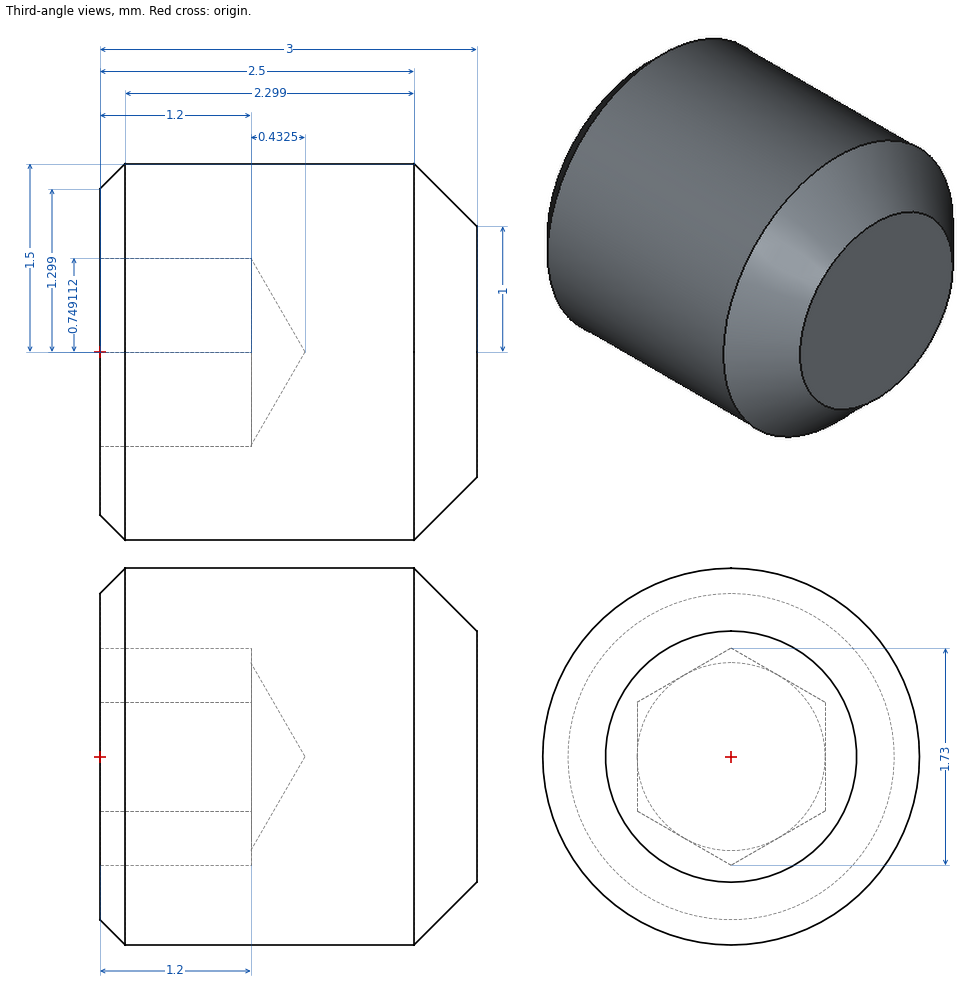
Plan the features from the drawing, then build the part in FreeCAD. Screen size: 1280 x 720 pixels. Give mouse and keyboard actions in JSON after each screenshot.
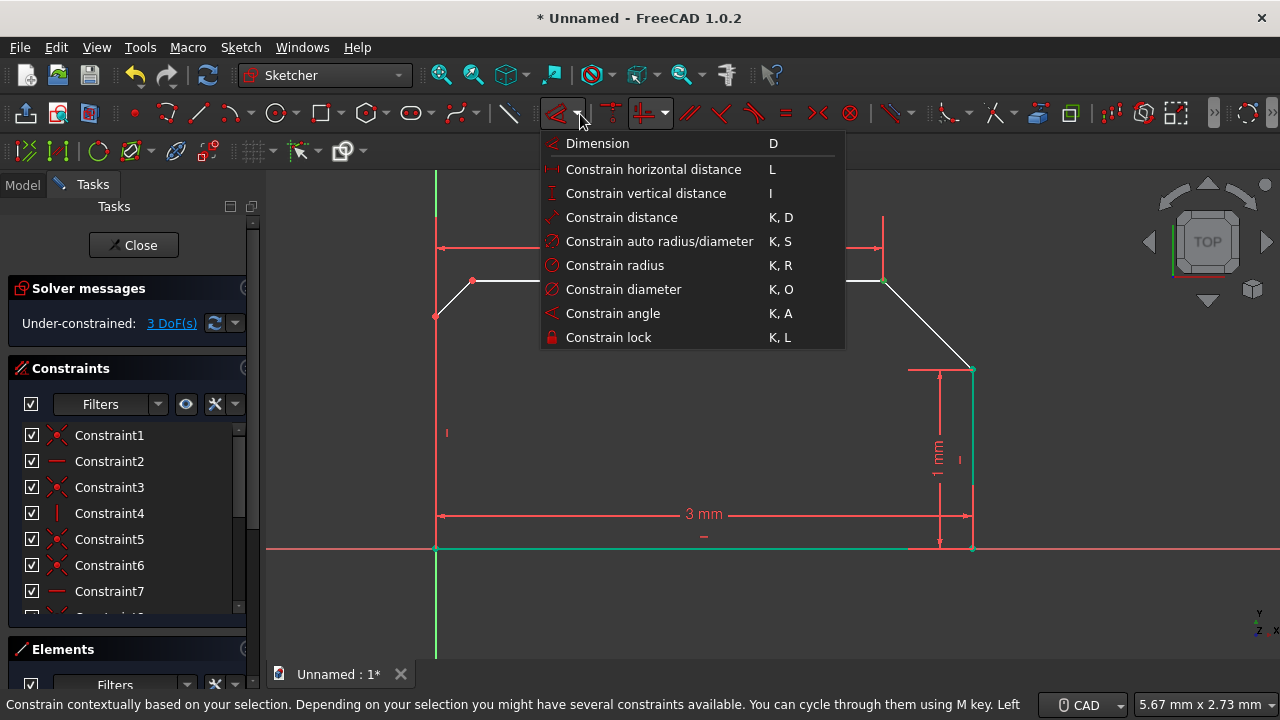
{"action": "left_click", "coordinate": [693, 193]}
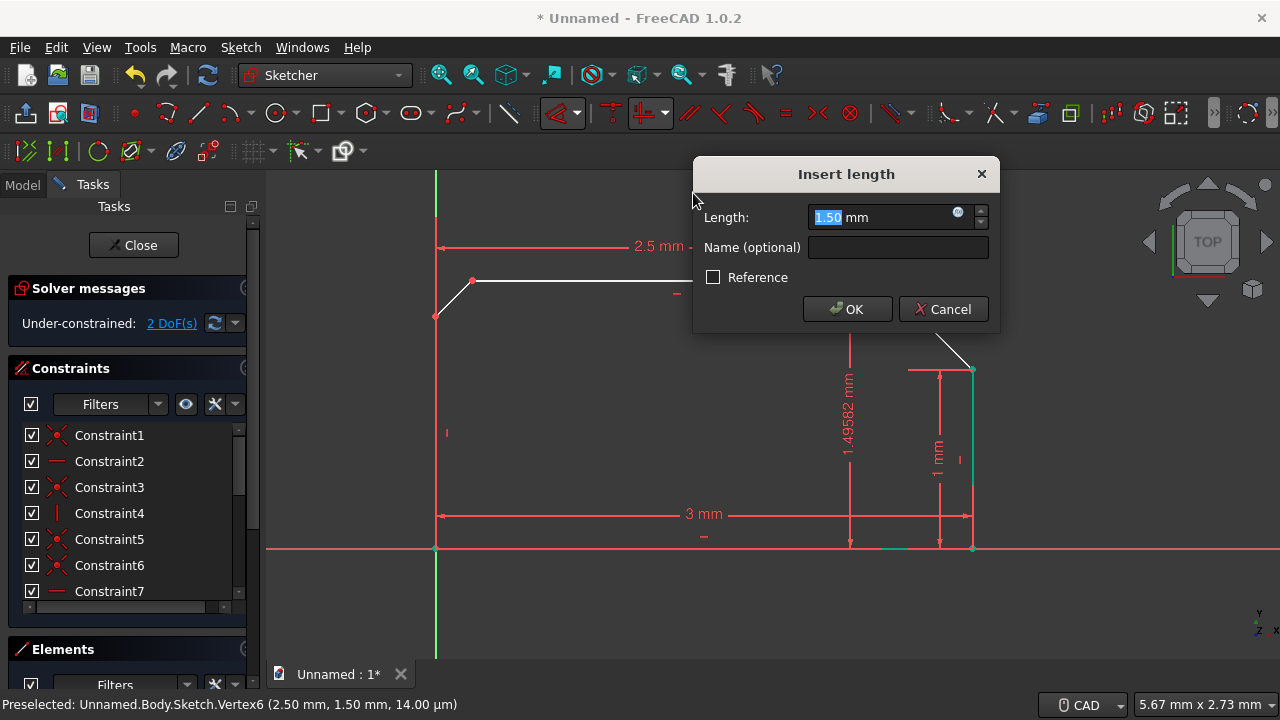
{"action": "type", "text": "1.5"}
{"action": "key", "text": "Return"}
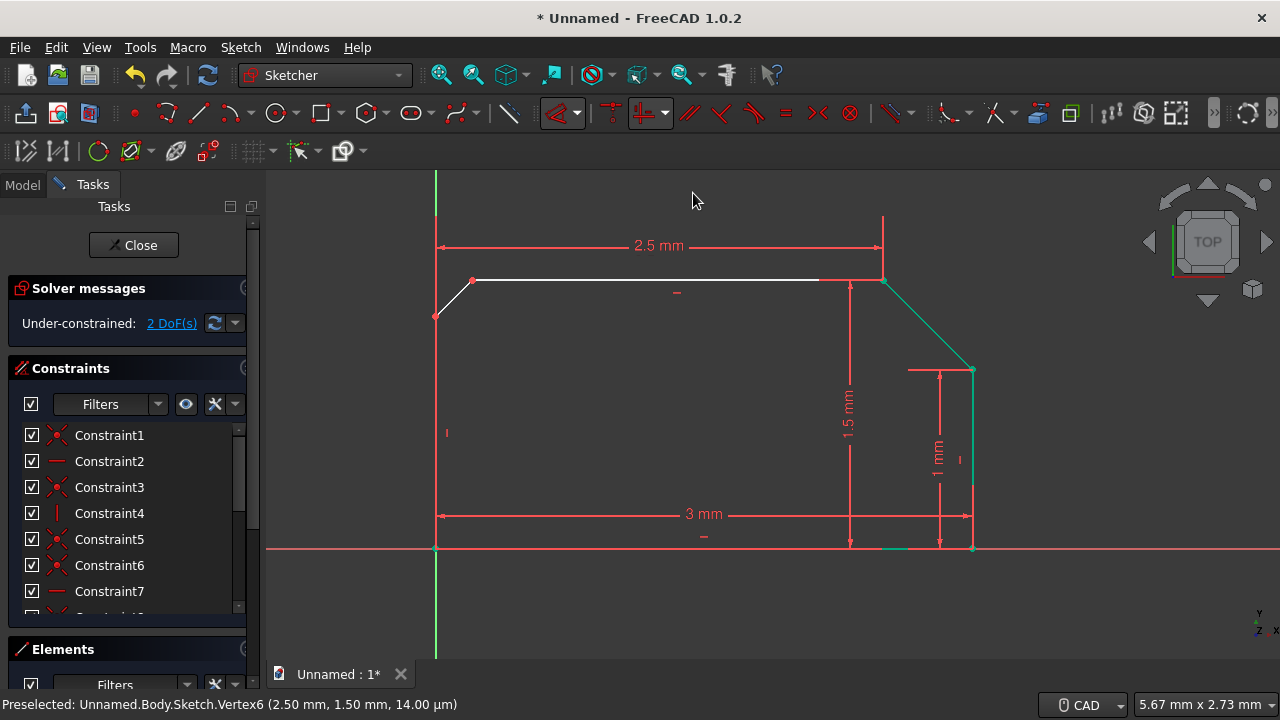
{"action": "left_click", "coordinate": [760, 280]}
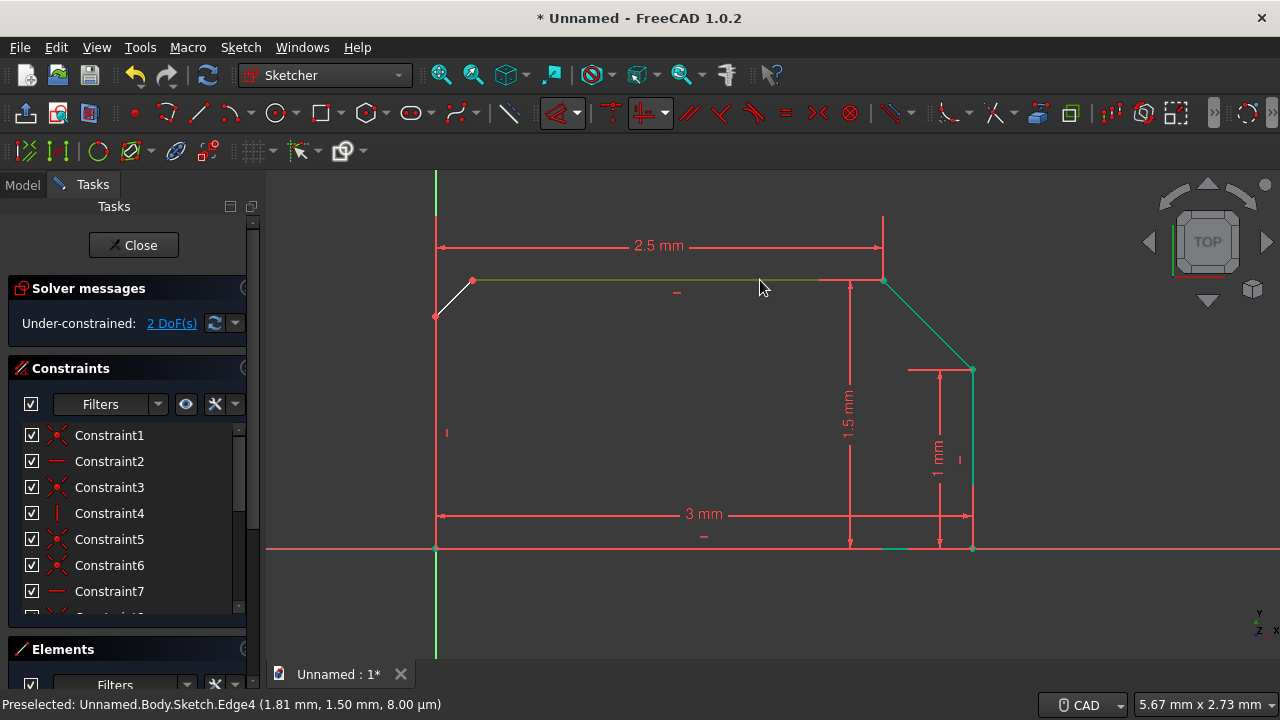
{"action": "key", "text": "l"}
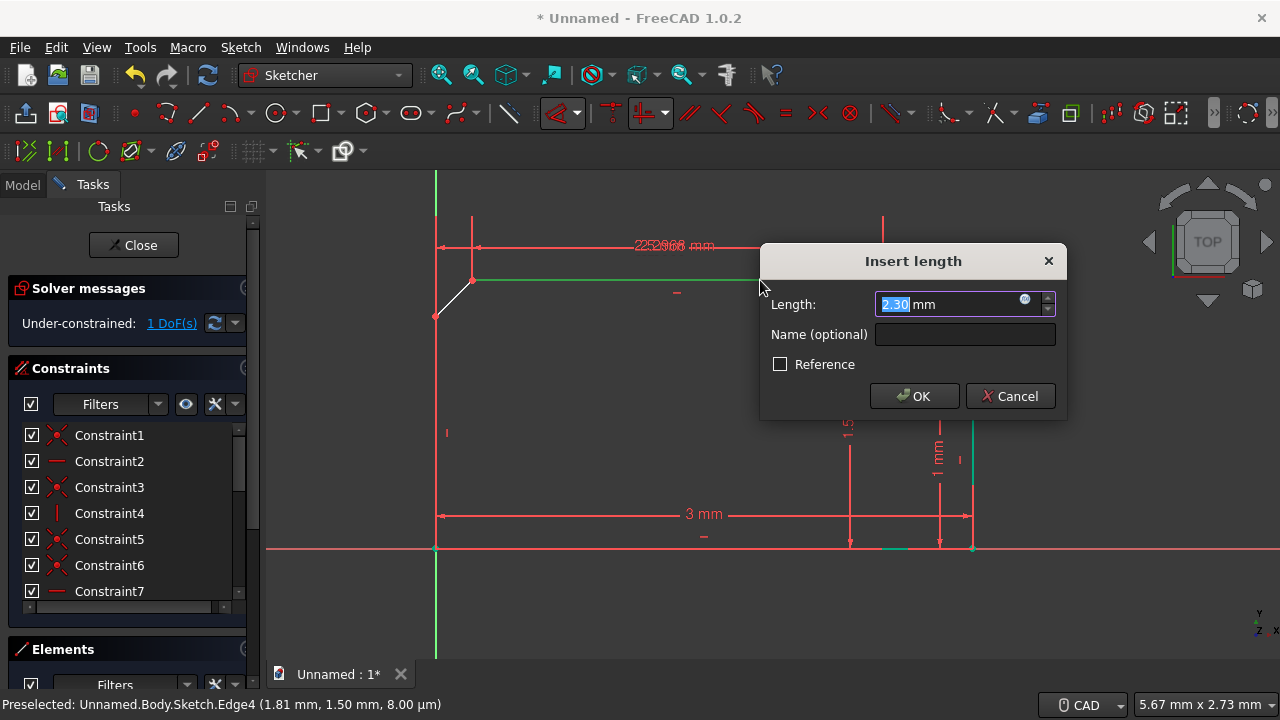
{"action": "type", "text": "2.299"}
{"action": "key", "text": "Return"}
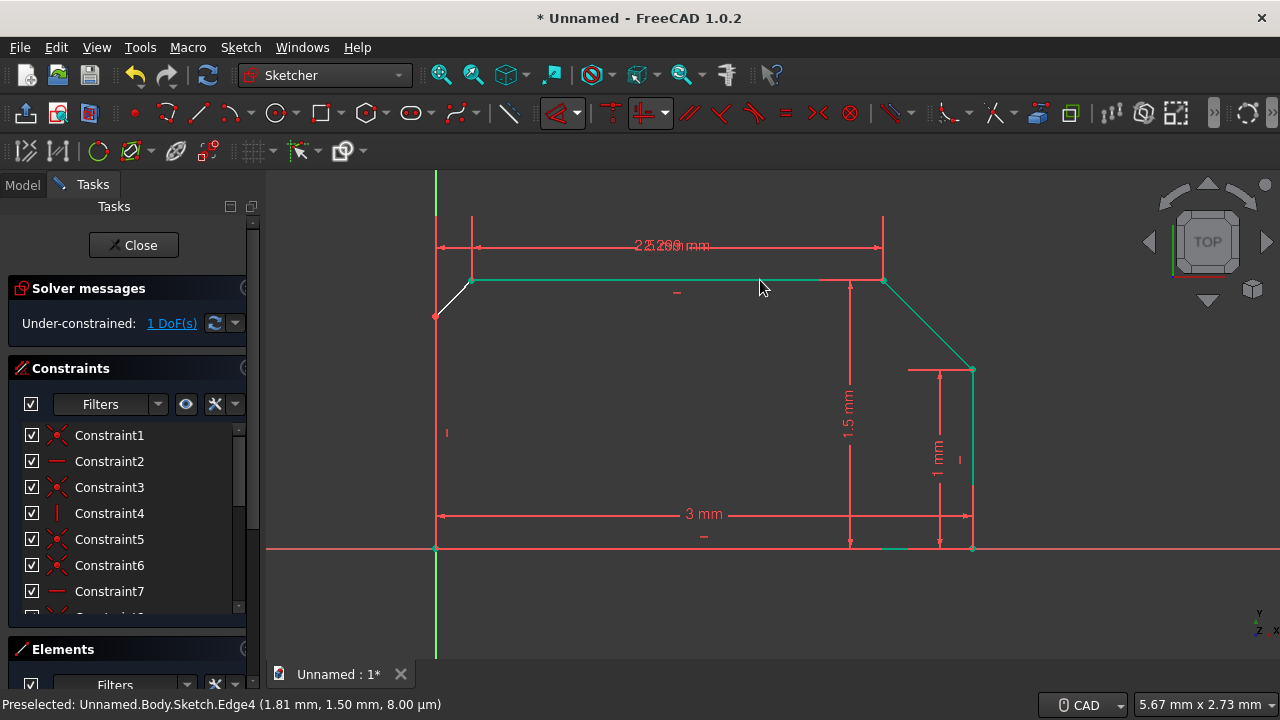
{"action": "left_click", "coordinate": [436, 387]}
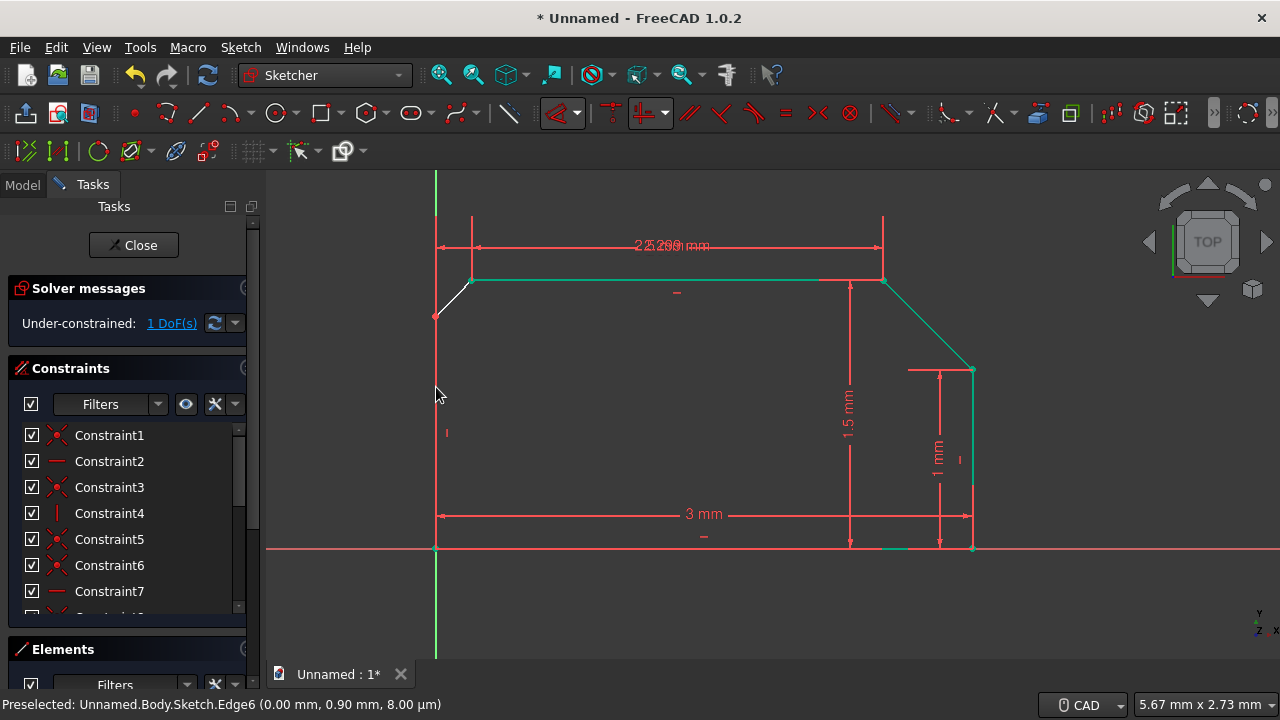
{"action": "left_click", "coordinate": [580, 114]}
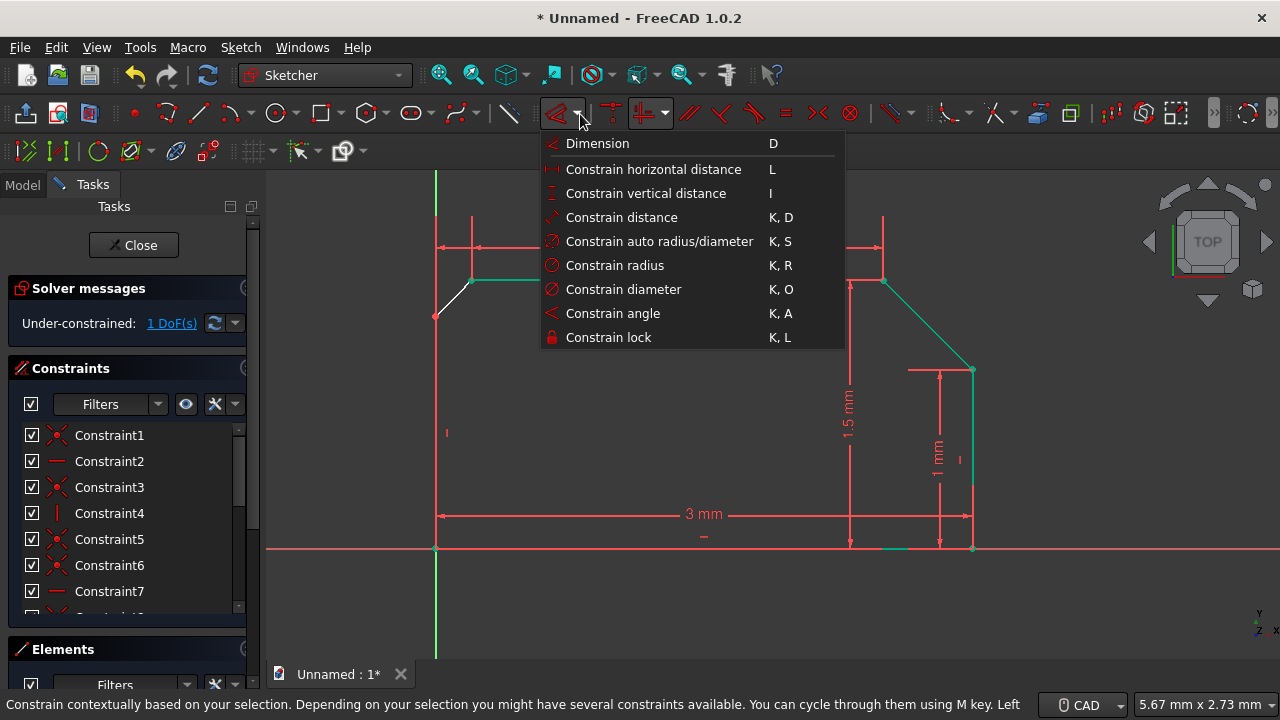
{"action": "left_click", "coordinate": [693, 193]}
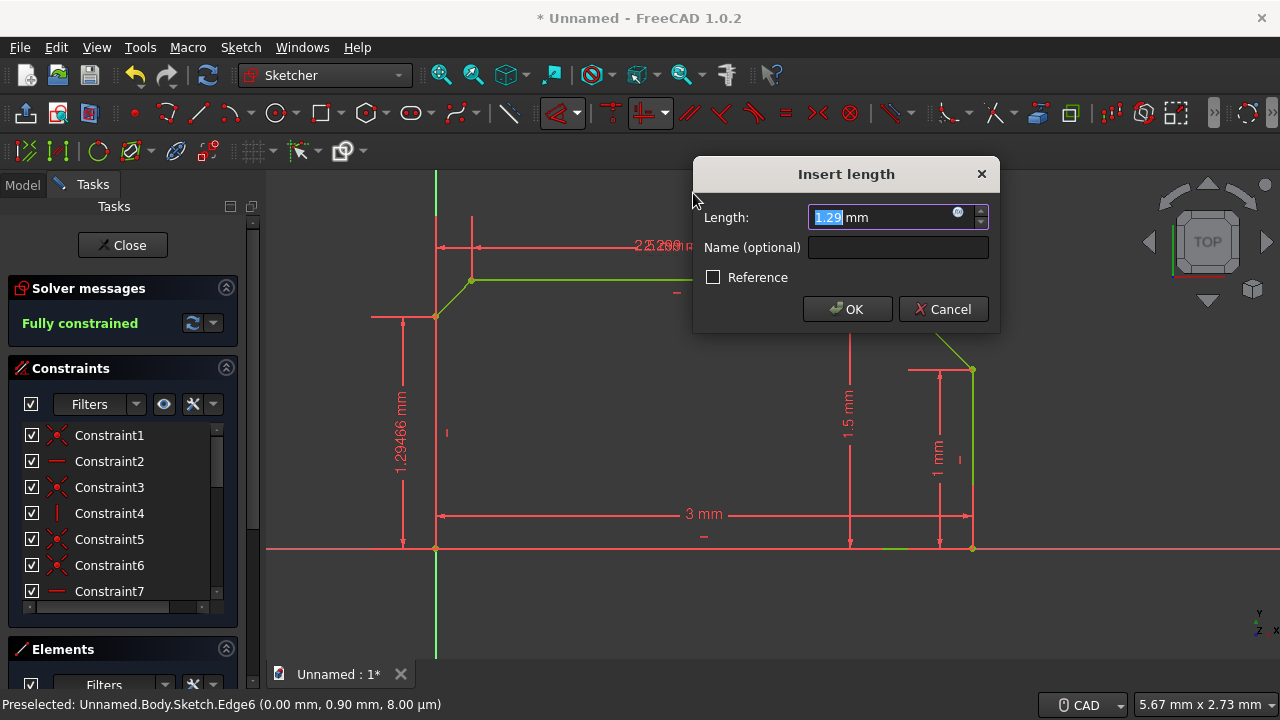
{"action": "type", "text": "1.299"}
{"action": "key", "text": "Return"}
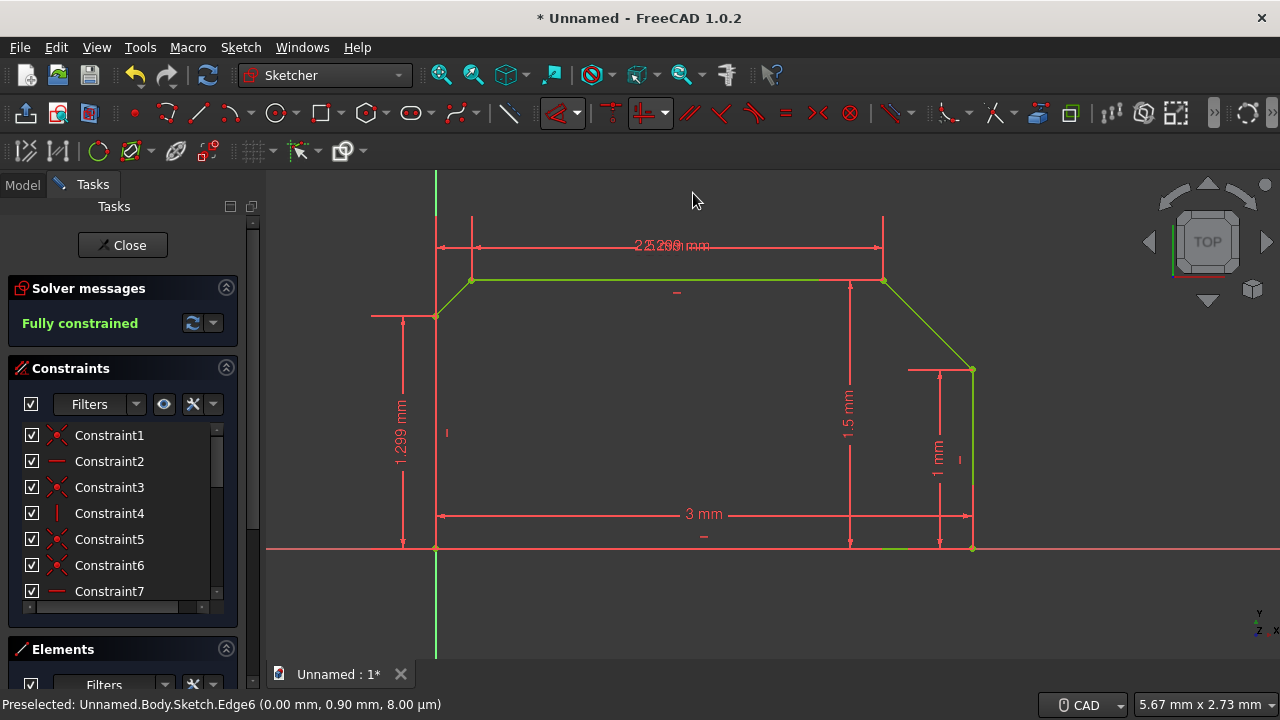
{"action": "left_click", "coordinate": [123, 245]}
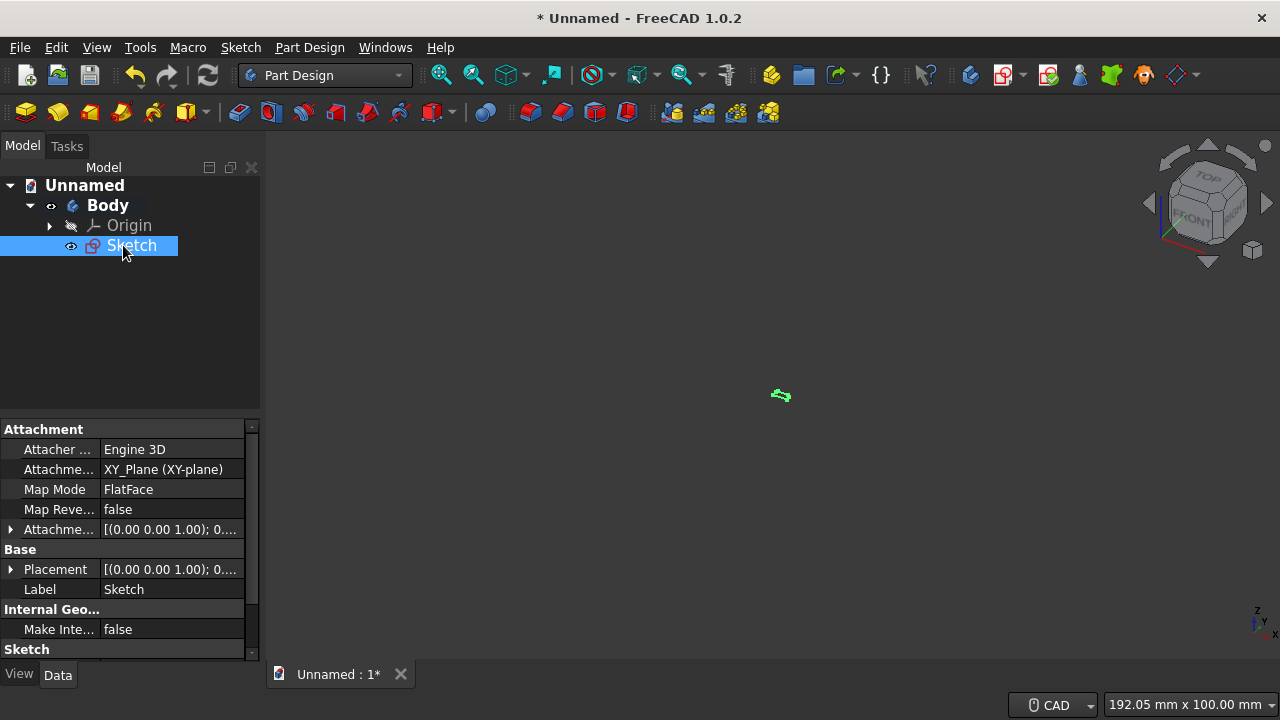
{"action": "left_click", "coordinate": [58, 112]}